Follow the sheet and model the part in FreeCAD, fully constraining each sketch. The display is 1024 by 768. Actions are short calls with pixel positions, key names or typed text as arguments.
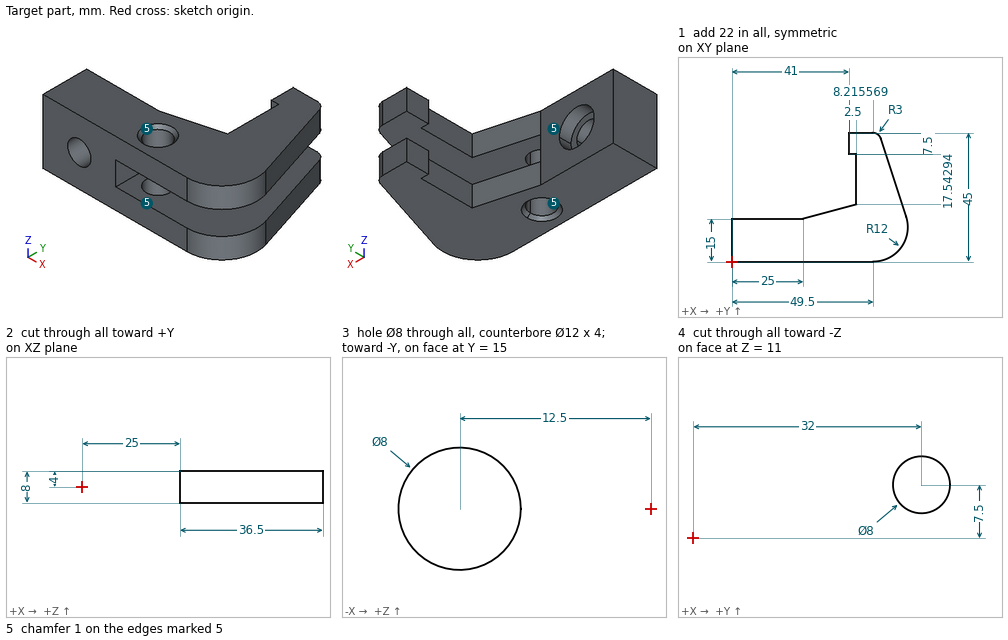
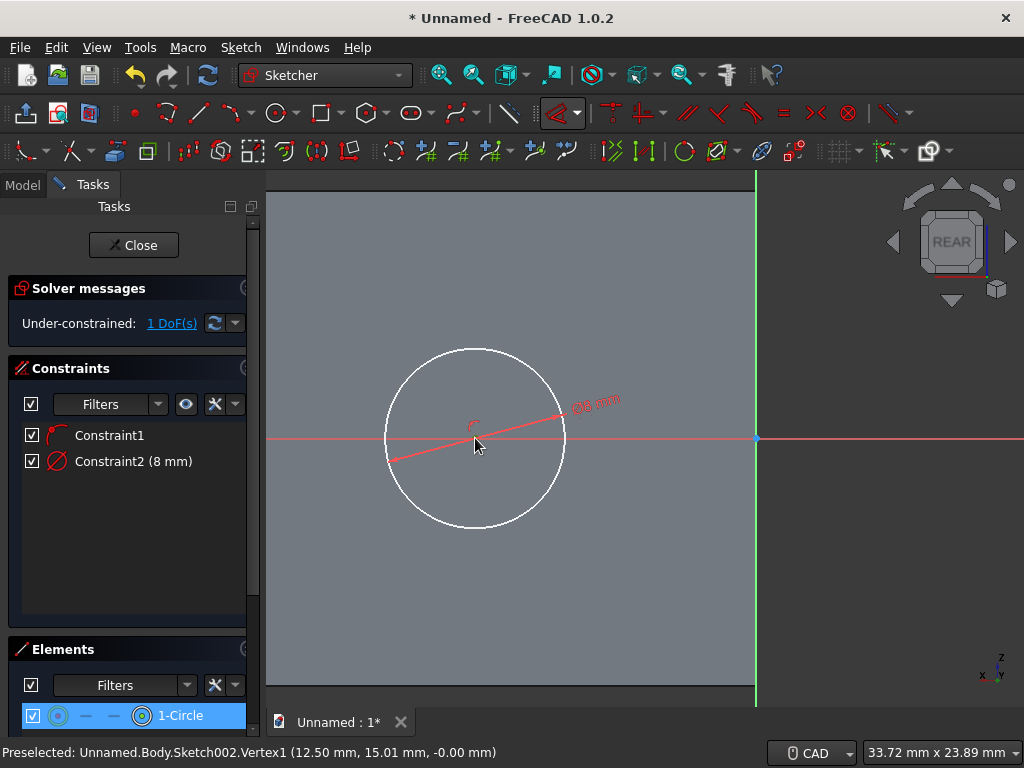
click(580, 114)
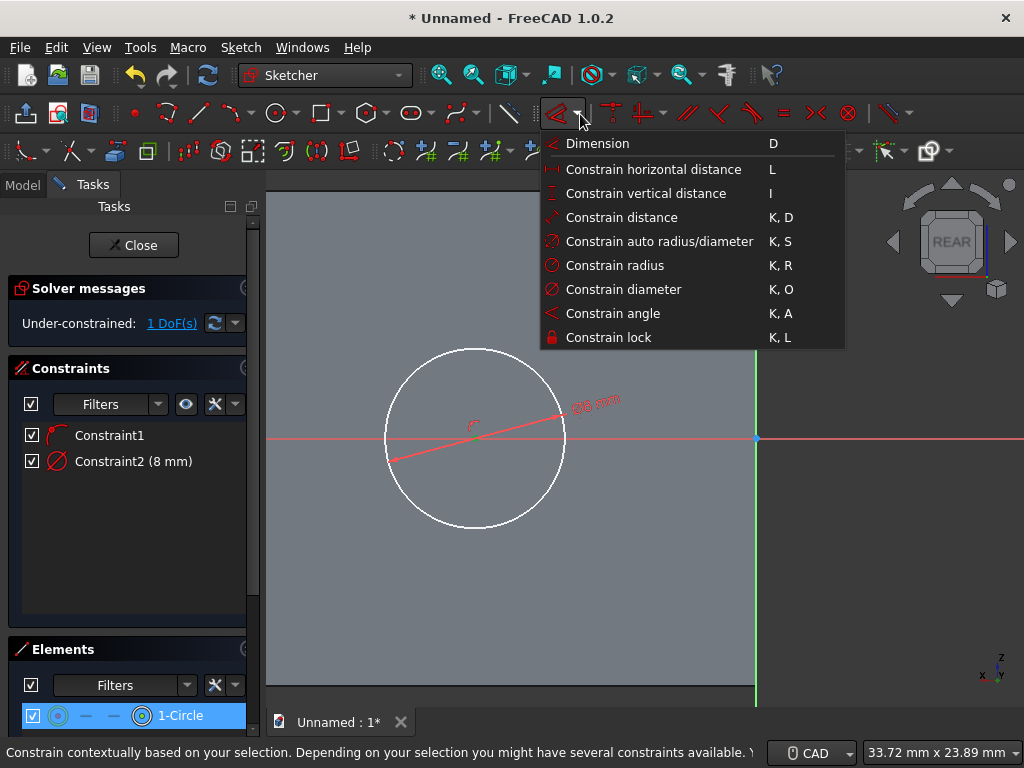
click(693, 169)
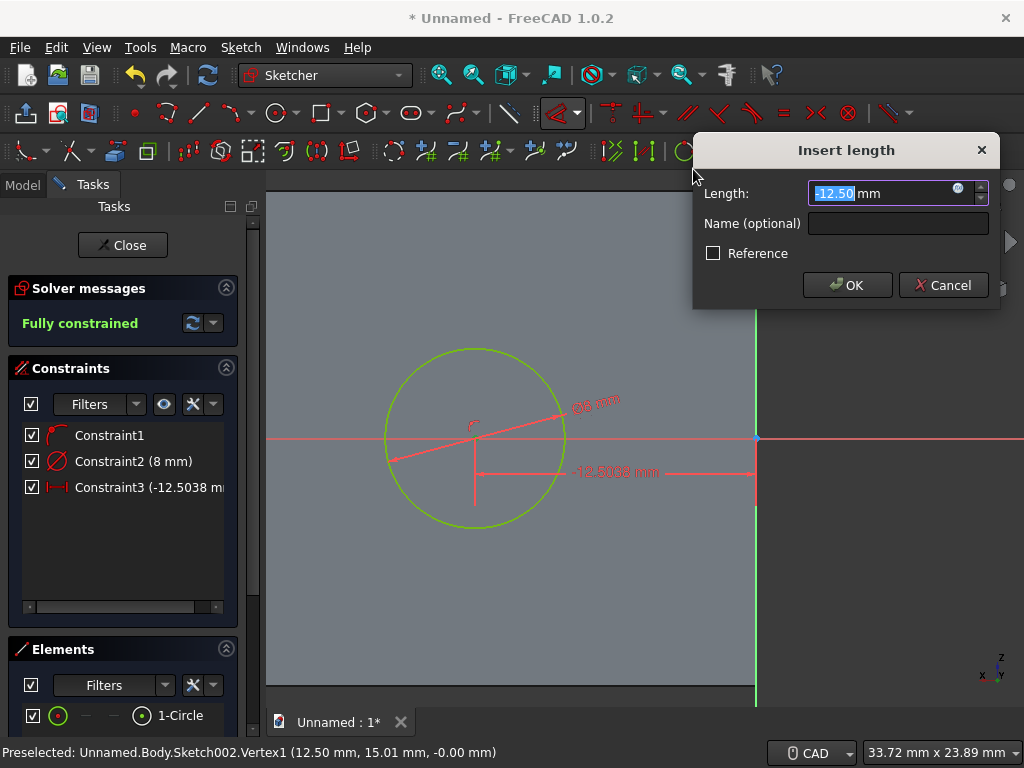
text(-12.5)
key(Return)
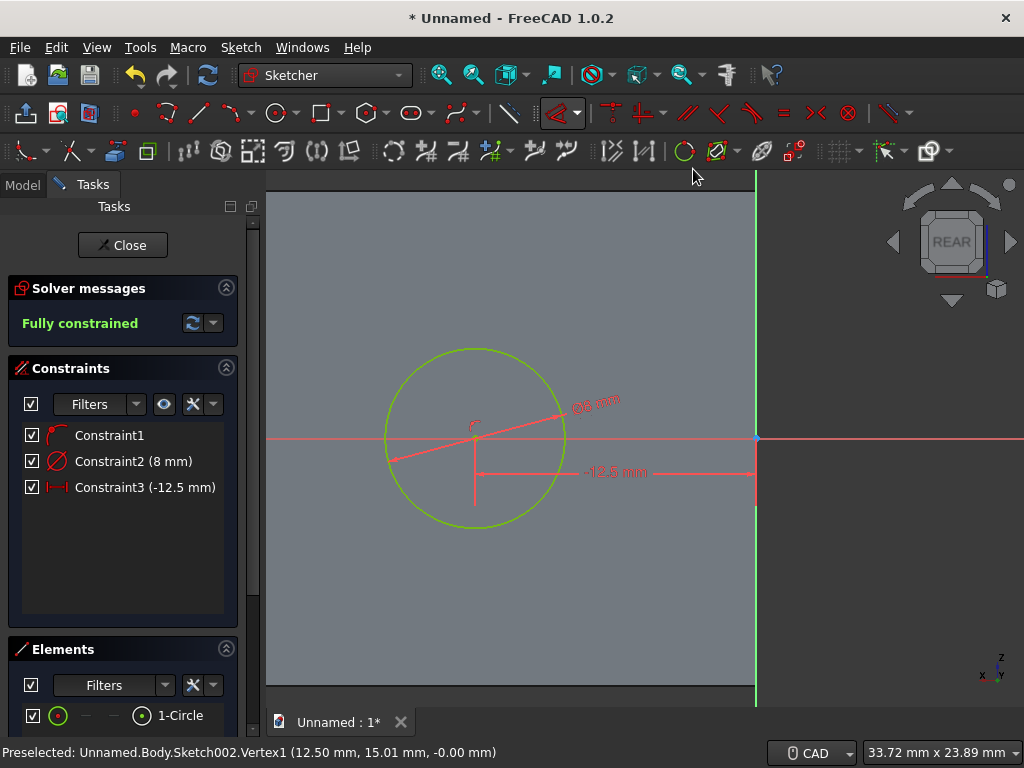
click(123, 245)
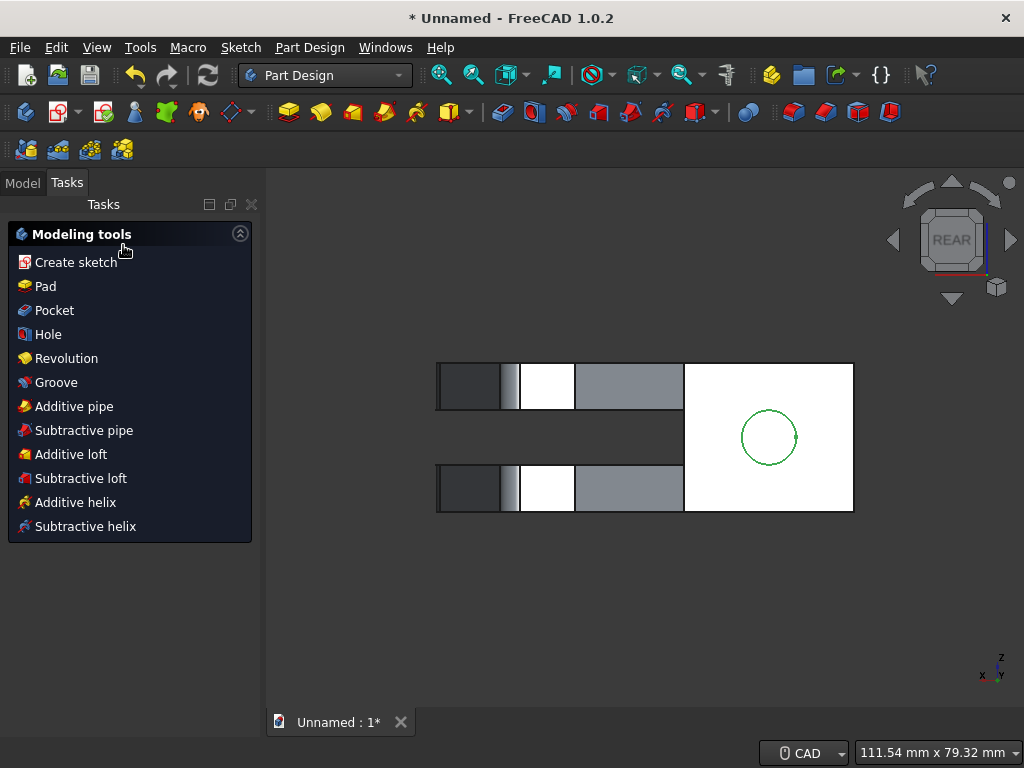
click(536, 112)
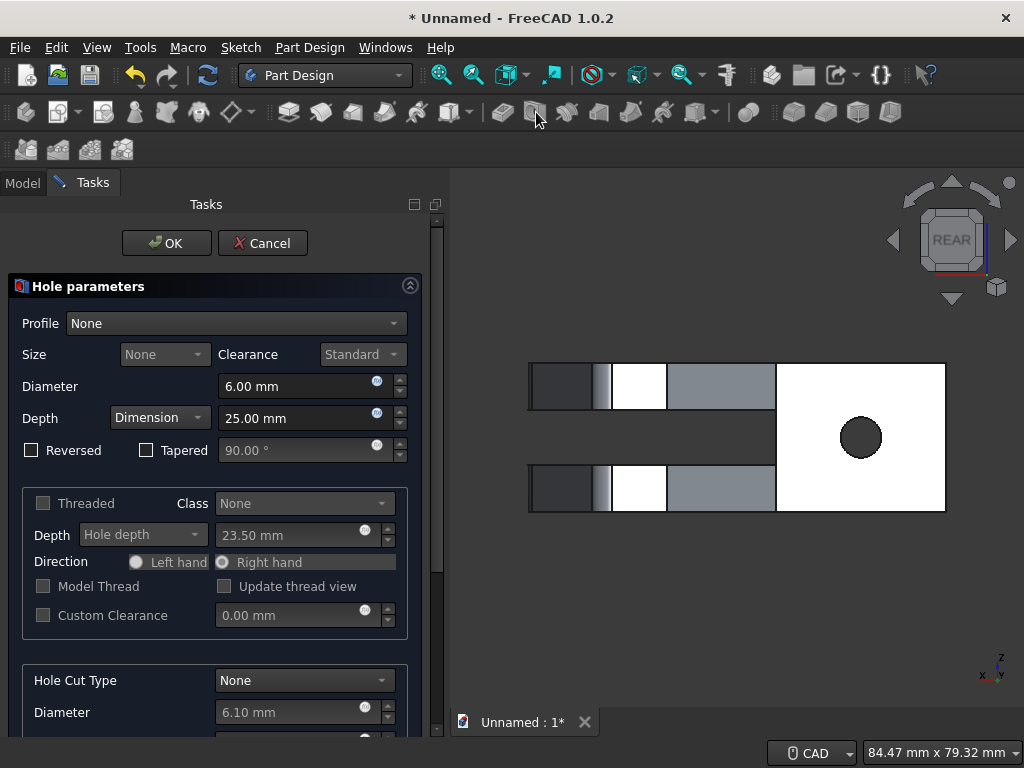
triple_click(305, 386)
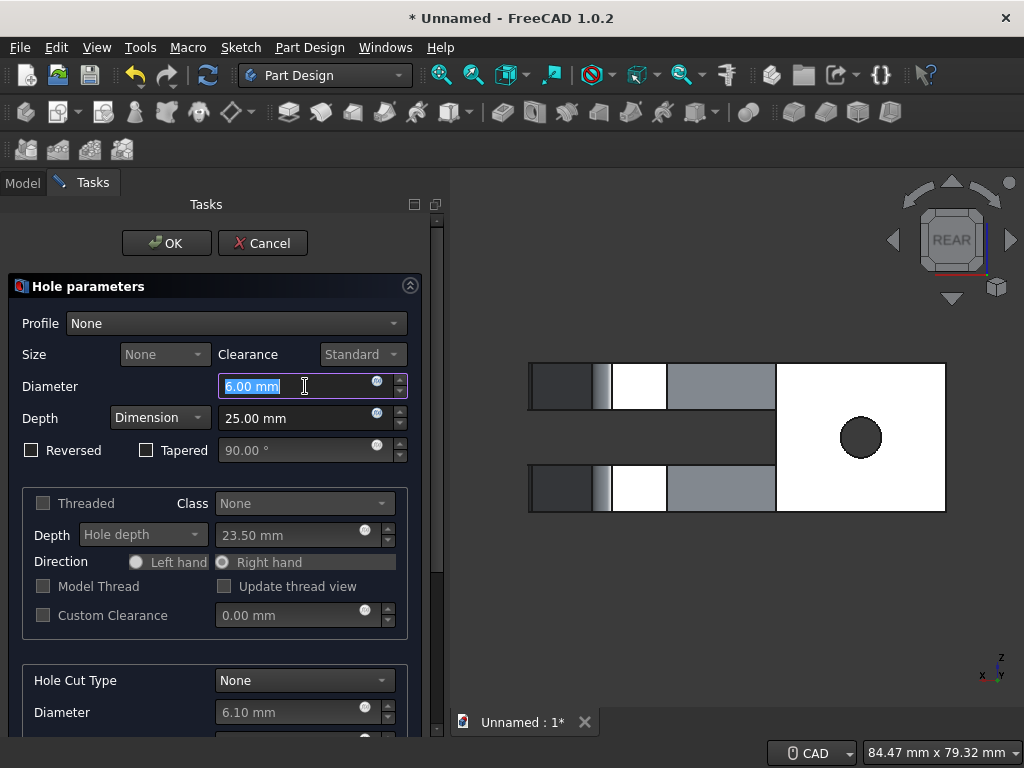
text(8)
key(Tab)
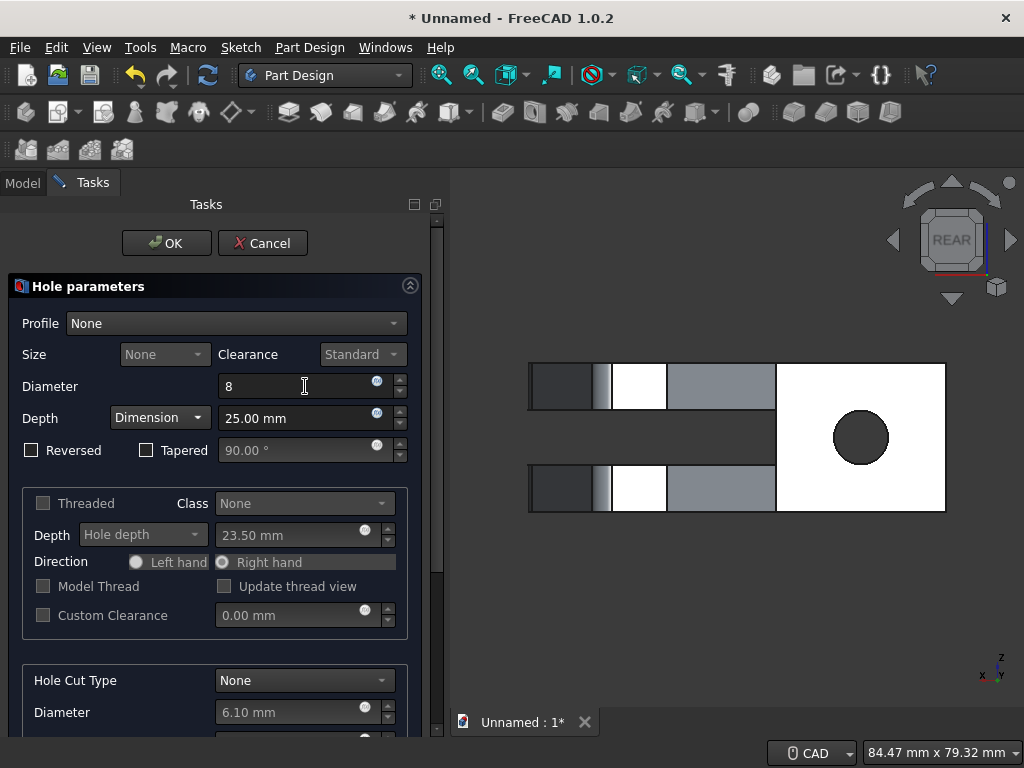
click(161, 418)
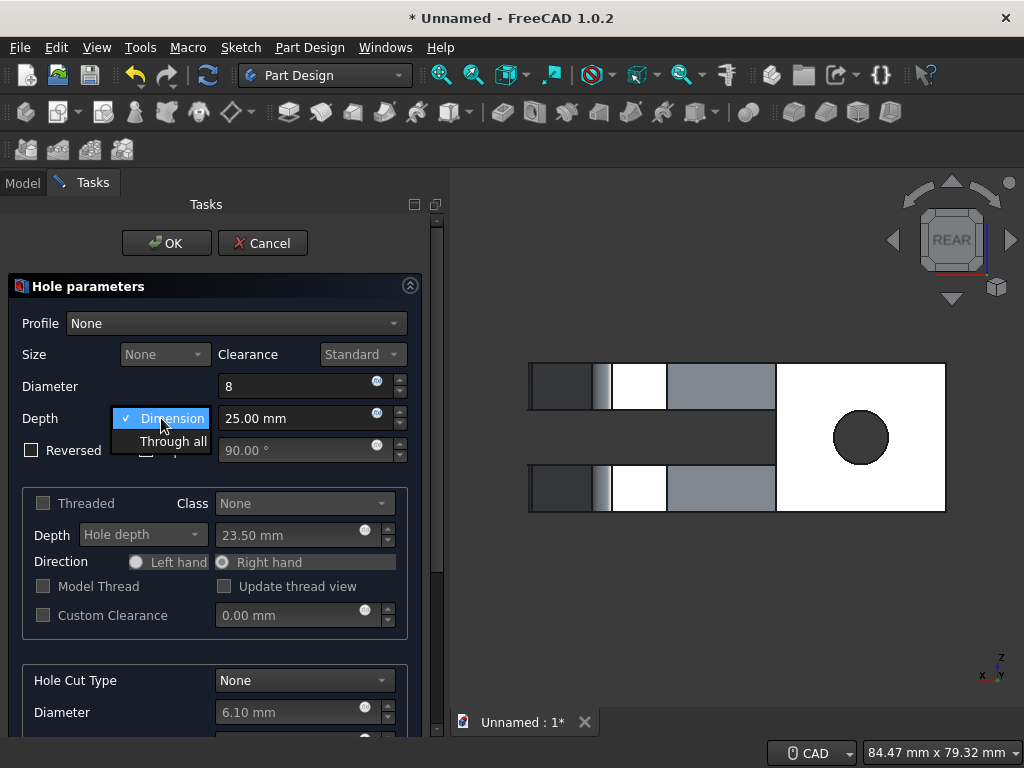
click(160, 442)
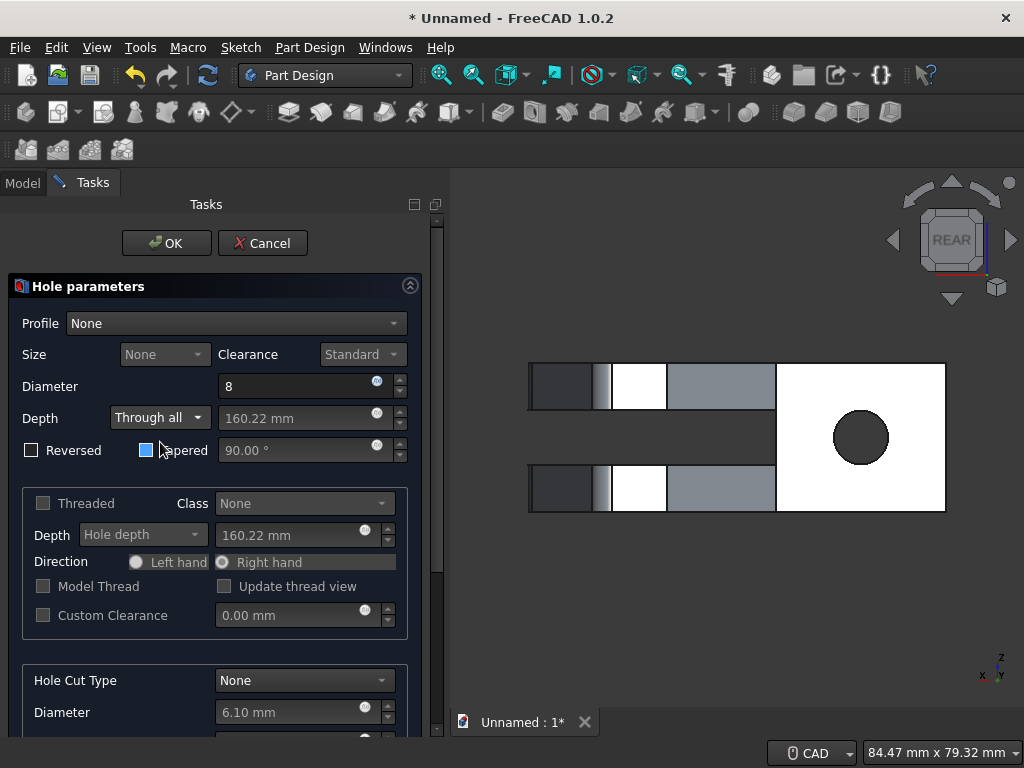
click(306, 680)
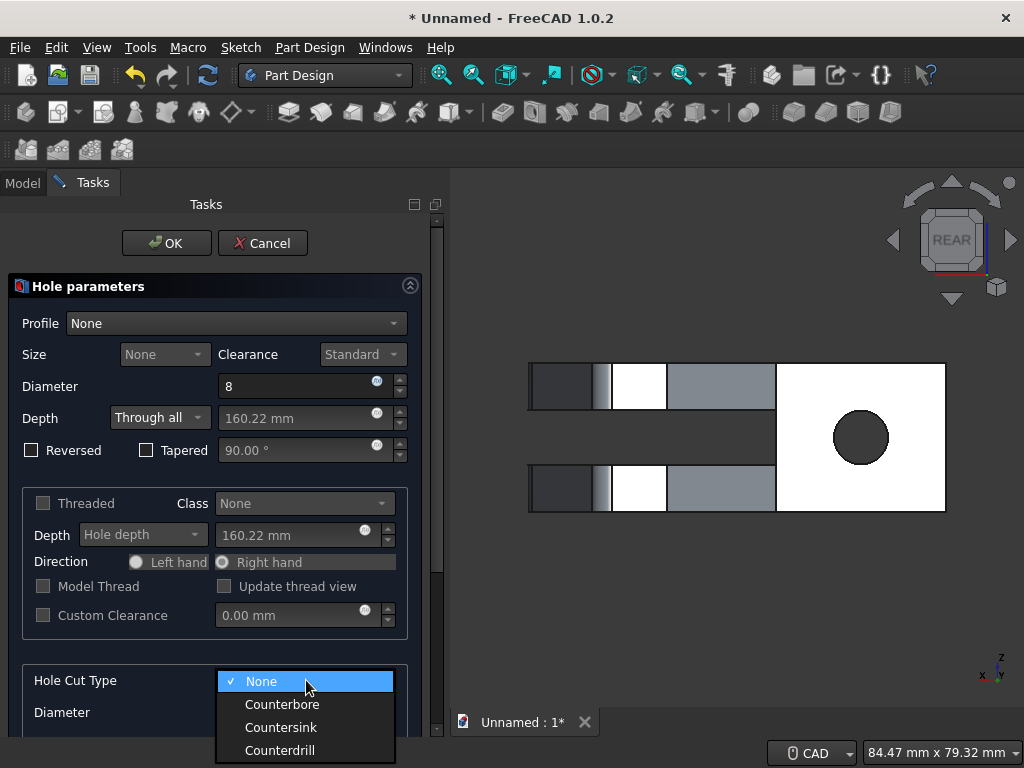
click(304, 704)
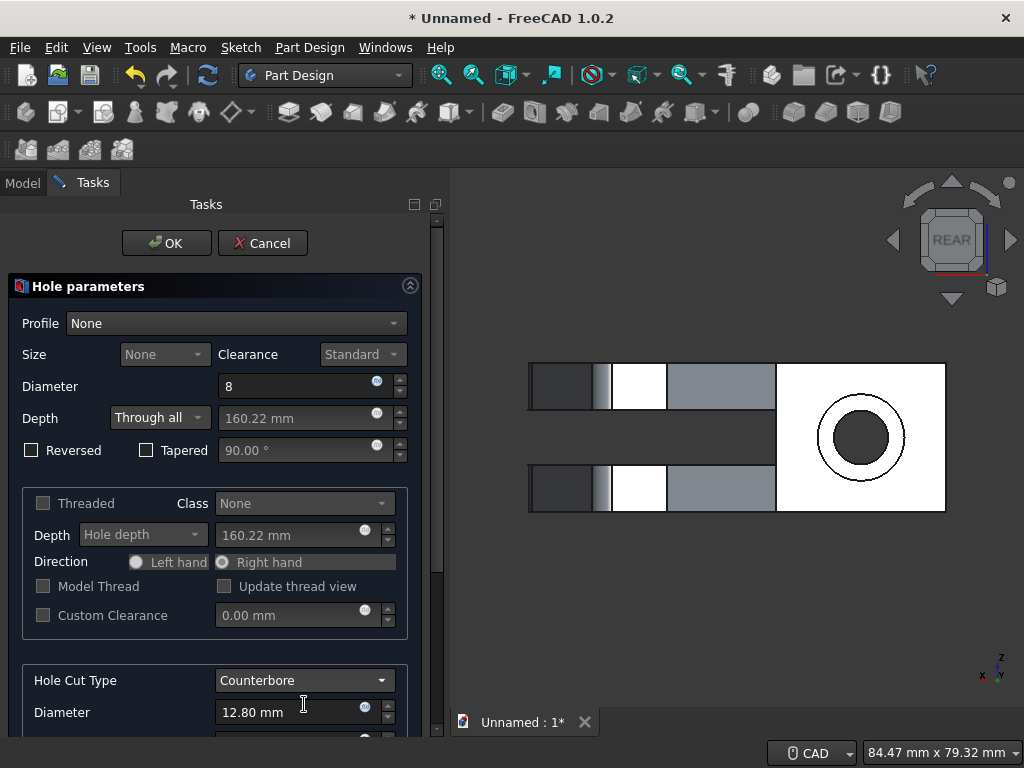
triple_click(298, 712)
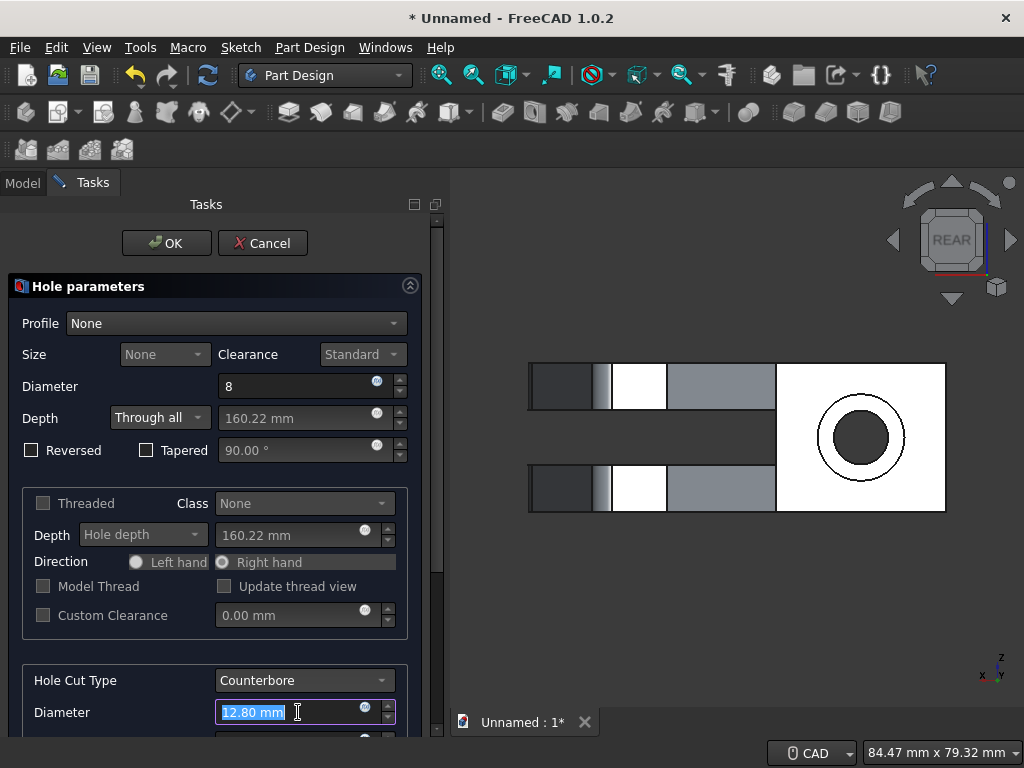
text(12)
key(Tab)